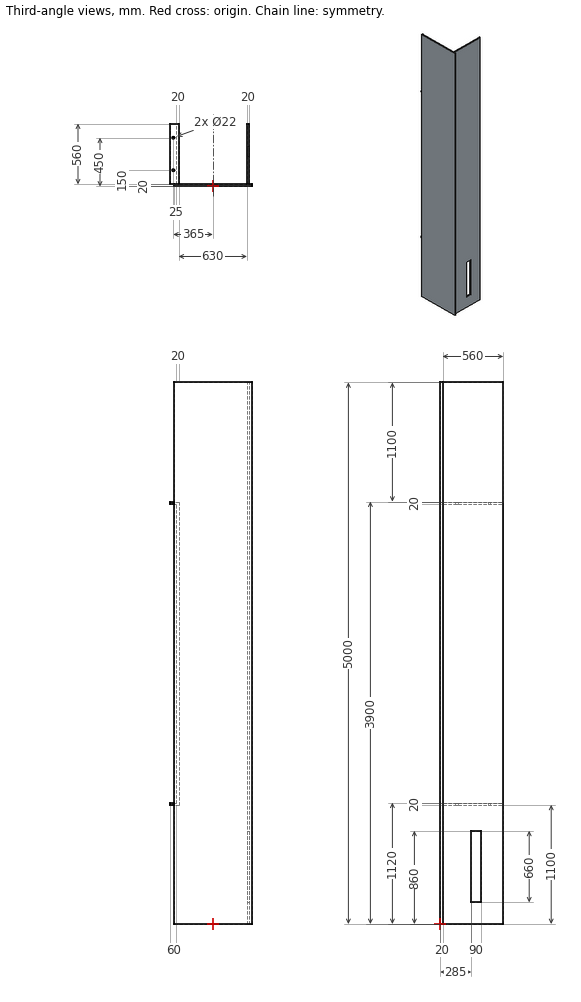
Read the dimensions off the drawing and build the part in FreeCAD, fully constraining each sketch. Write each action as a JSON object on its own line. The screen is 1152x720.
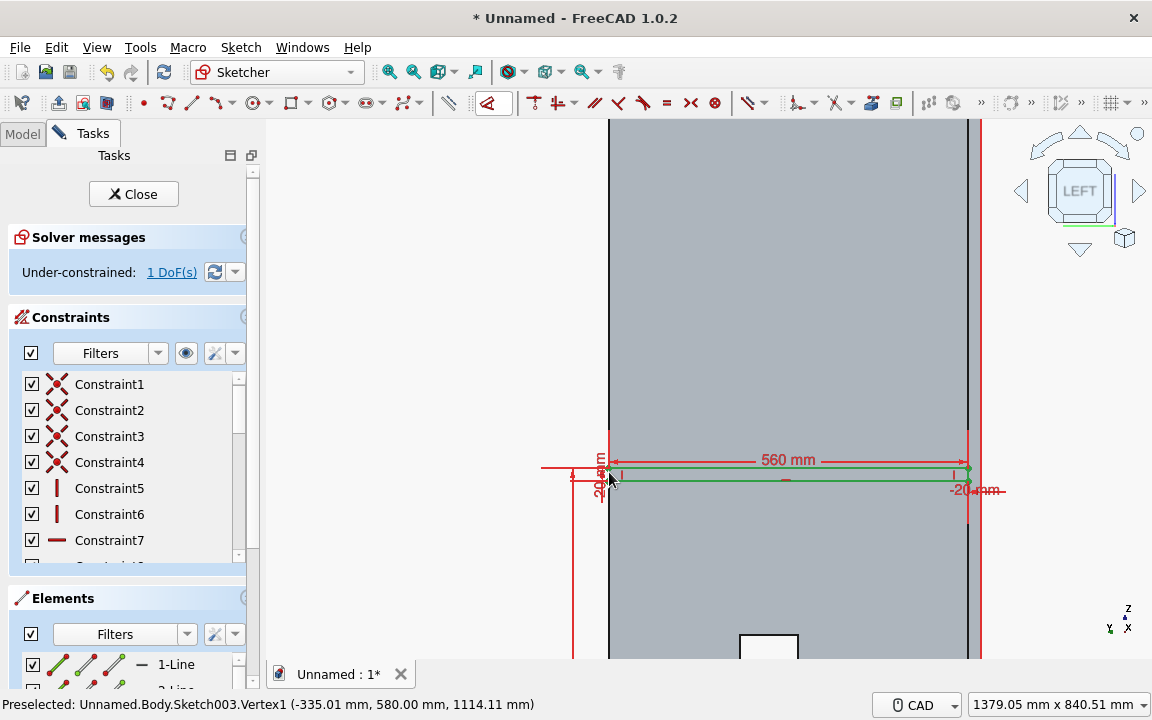
{"action": "scroll", "coordinate": [616, 460], "scroll_direction": "down", "scroll_amount": 10}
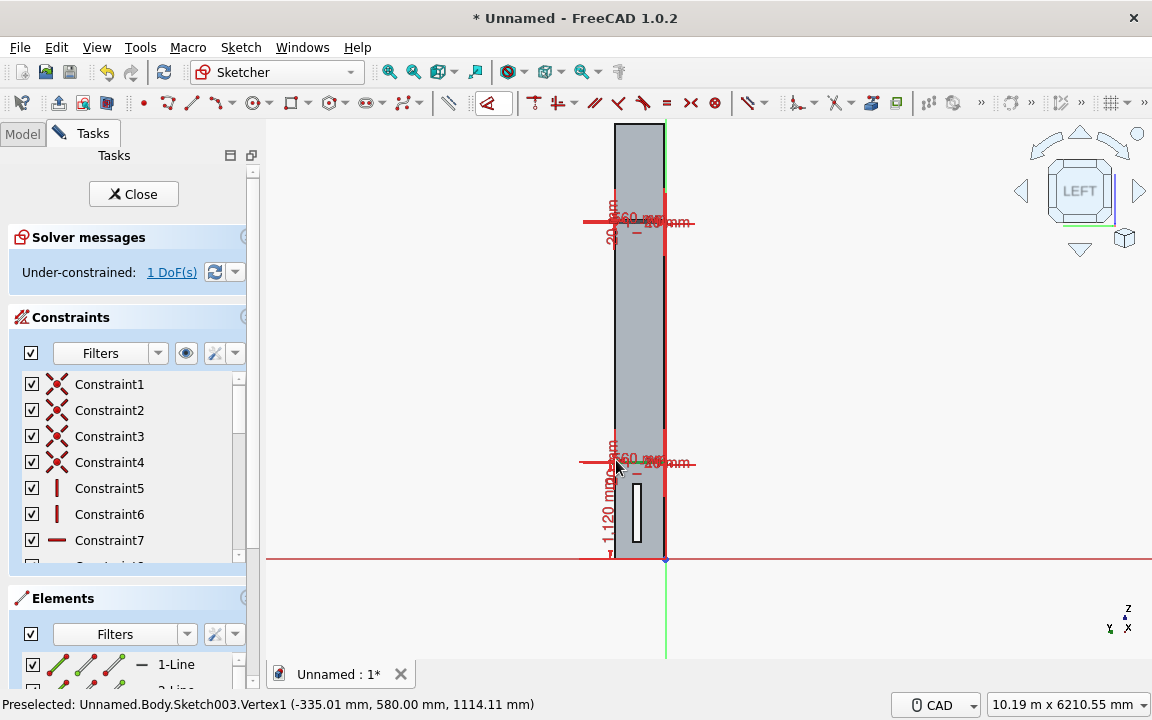
{"action": "scroll", "coordinate": [615, 221], "scroll_direction": "up", "scroll_amount": 10}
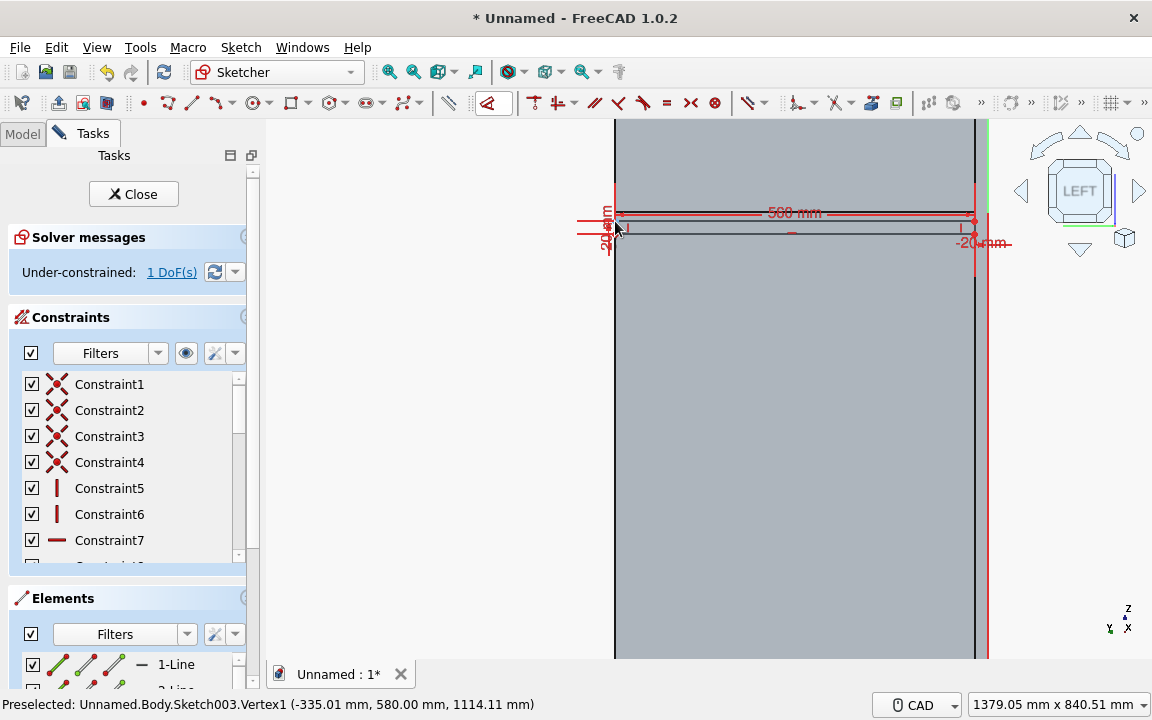
{"action": "left_click", "coordinate": [615, 221]}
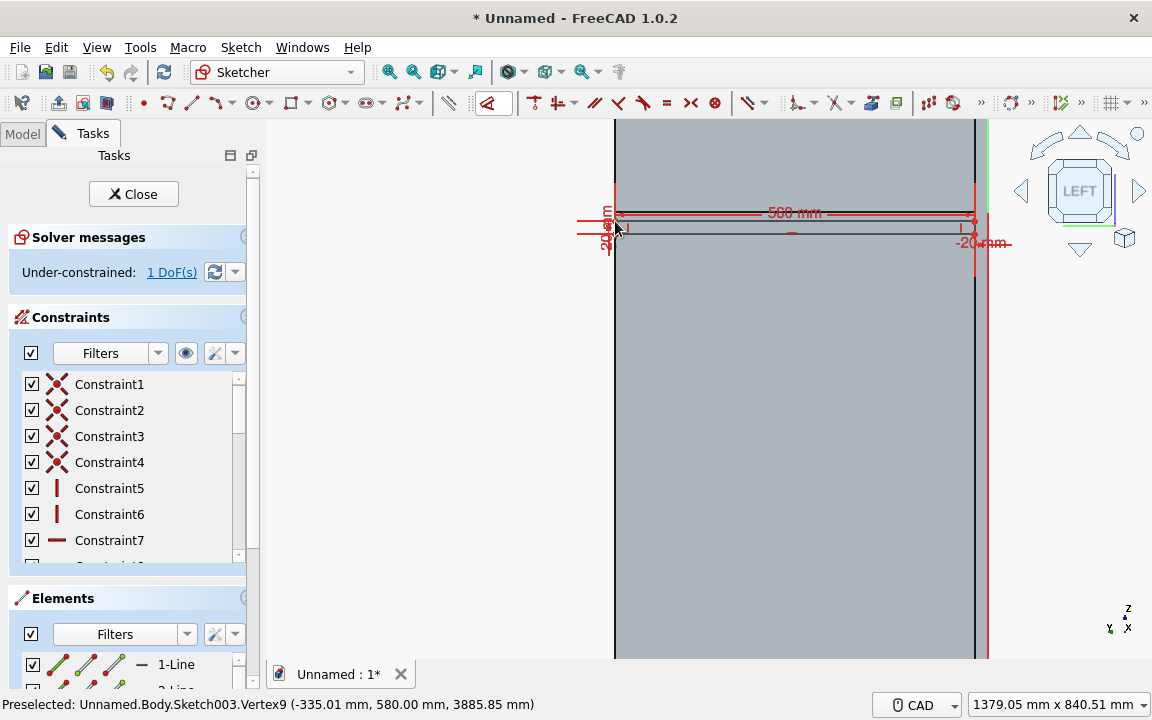
{"action": "left_click", "coordinate": [506, 104]}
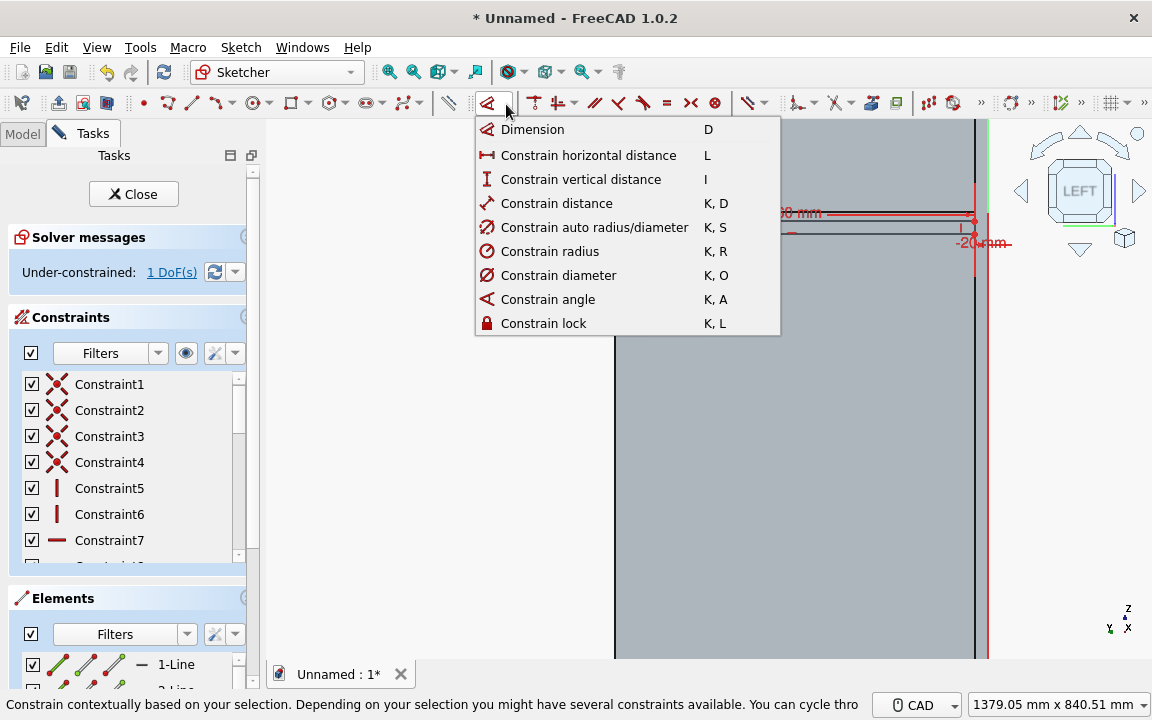
{"action": "left_click", "coordinate": [628, 179]}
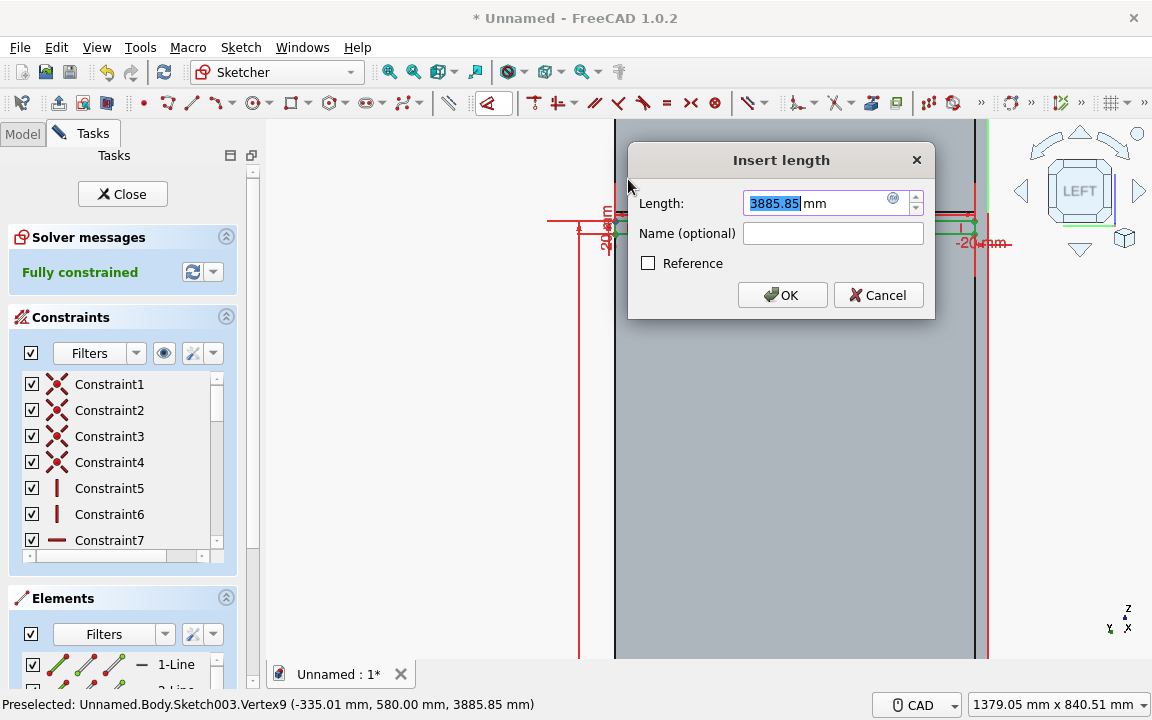
{"action": "type", "text": "3900"}
{"action": "key", "text": "Return"}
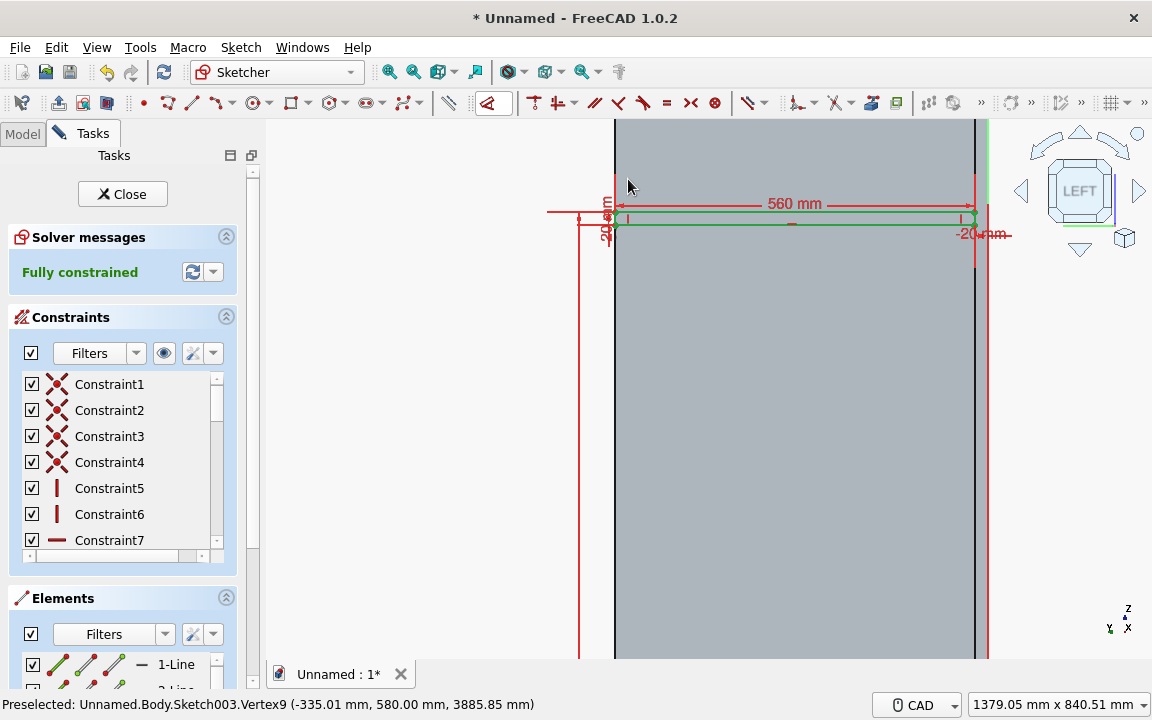
{"action": "left_click", "coordinate": [123, 194]}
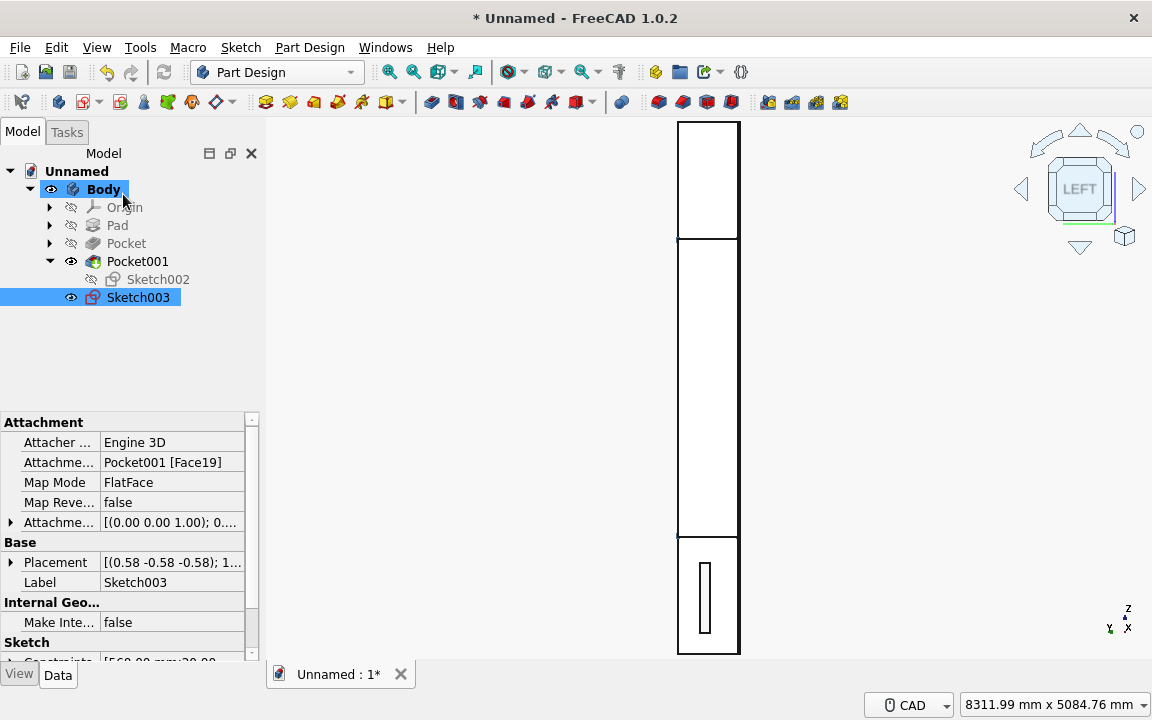
{"action": "left_click", "coordinate": [266, 102]}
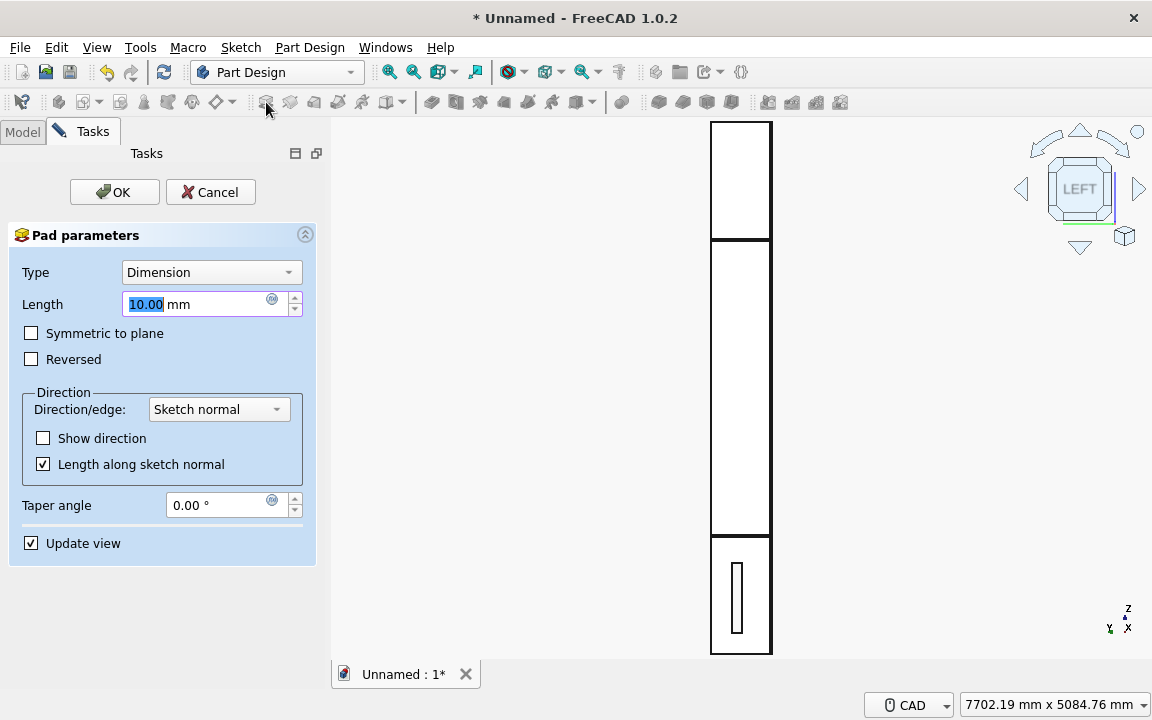
{"action": "type", "text": "60"}
{"action": "key", "text": "Tab"}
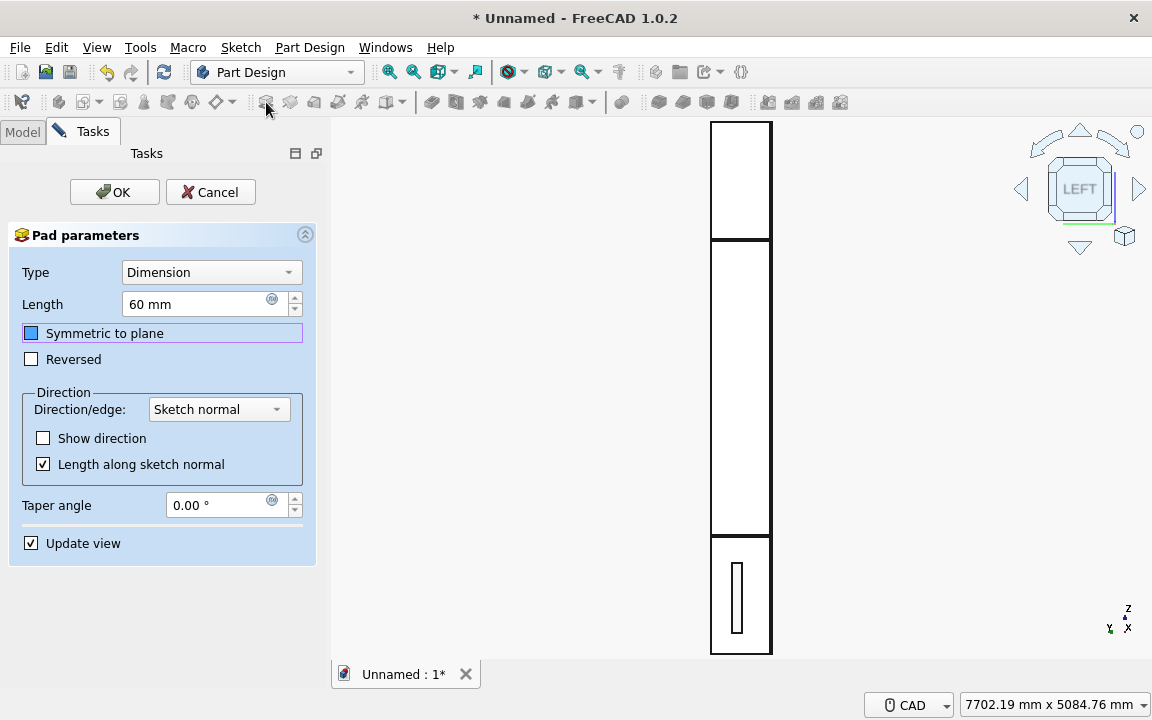
{"action": "left_click", "coordinate": [115, 192]}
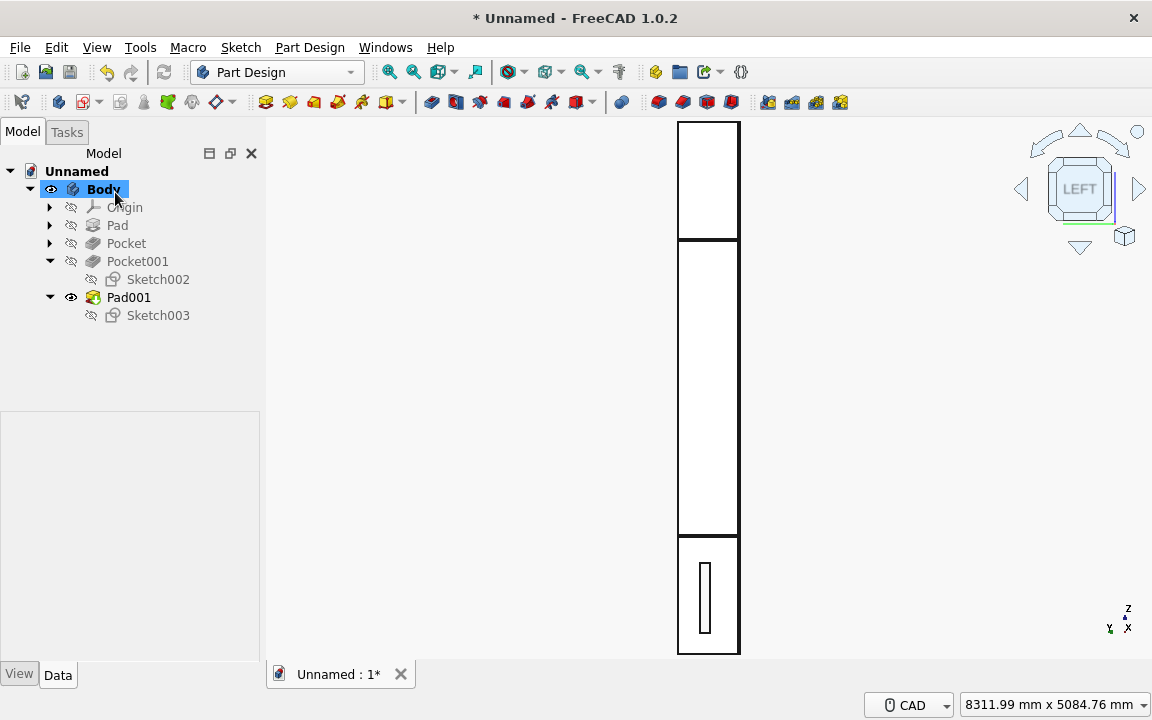
{"action": "key", "text": "0"}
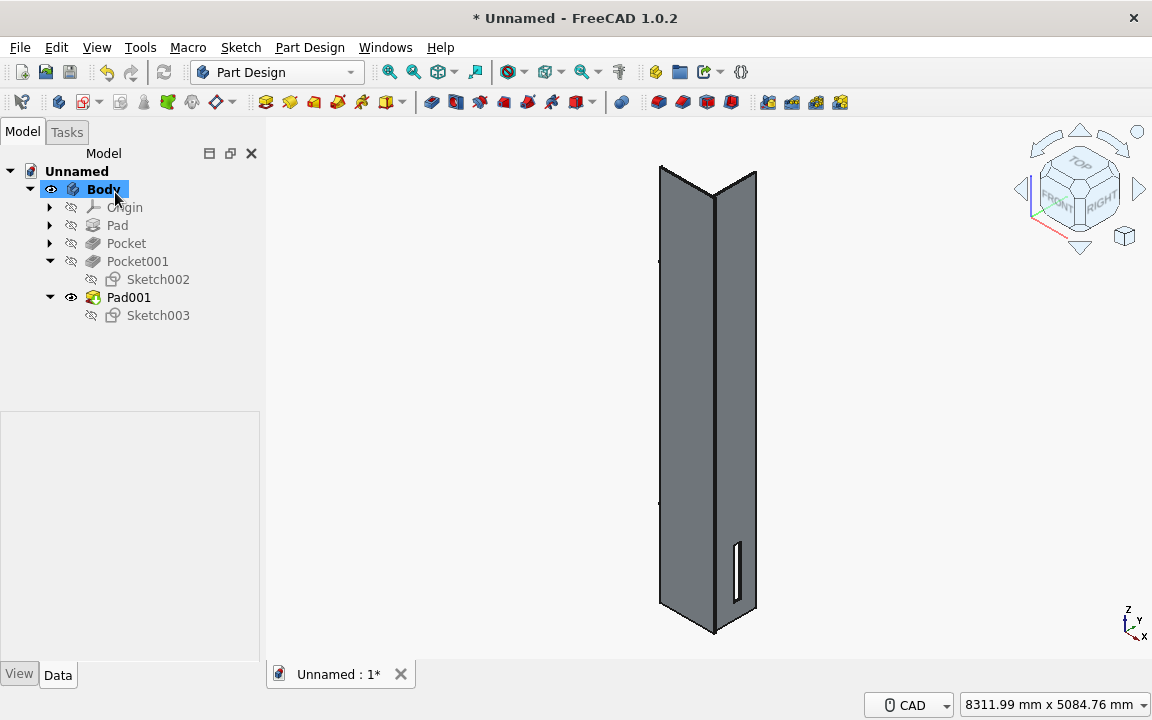
{"action": "scroll", "coordinate": [701, 239], "scroll_direction": "up", "scroll_amount": 6}